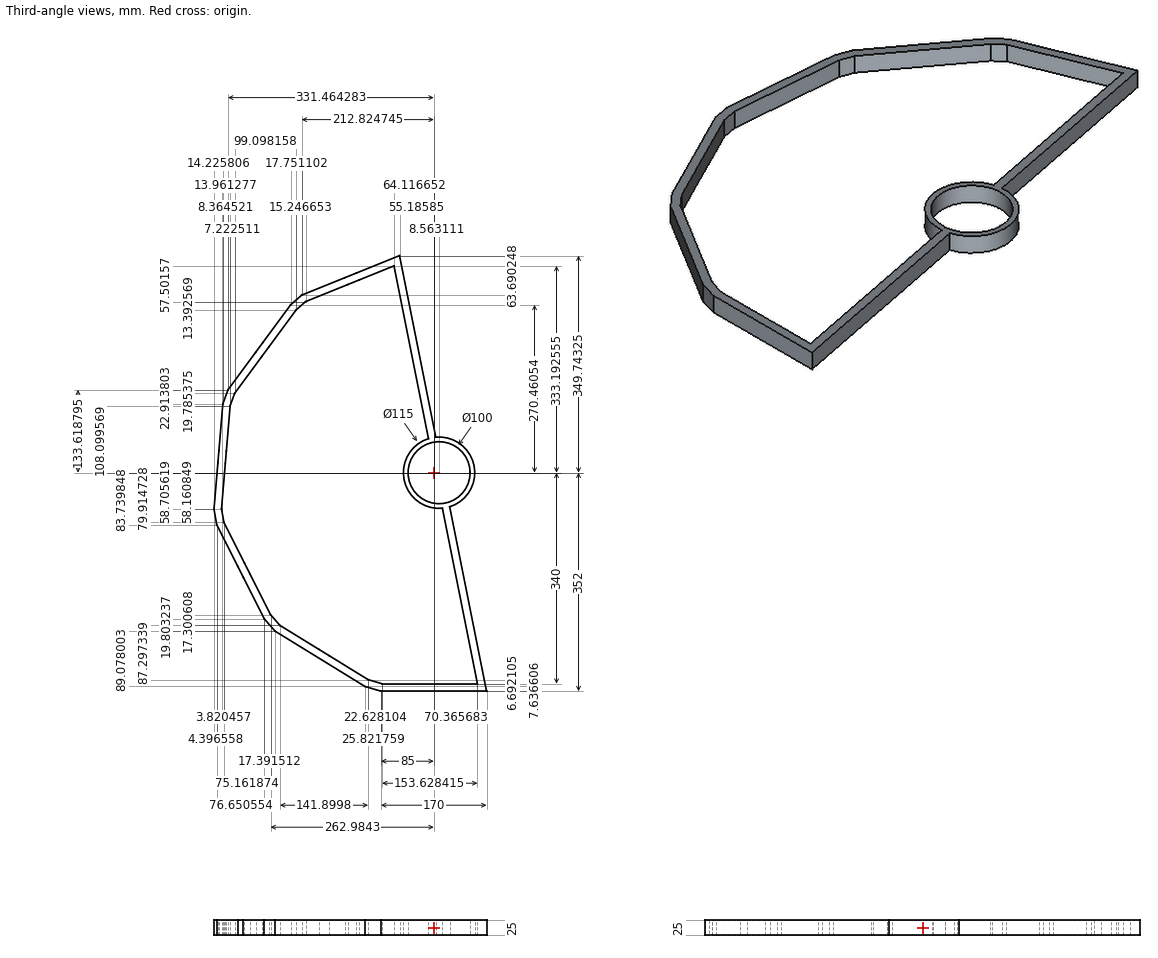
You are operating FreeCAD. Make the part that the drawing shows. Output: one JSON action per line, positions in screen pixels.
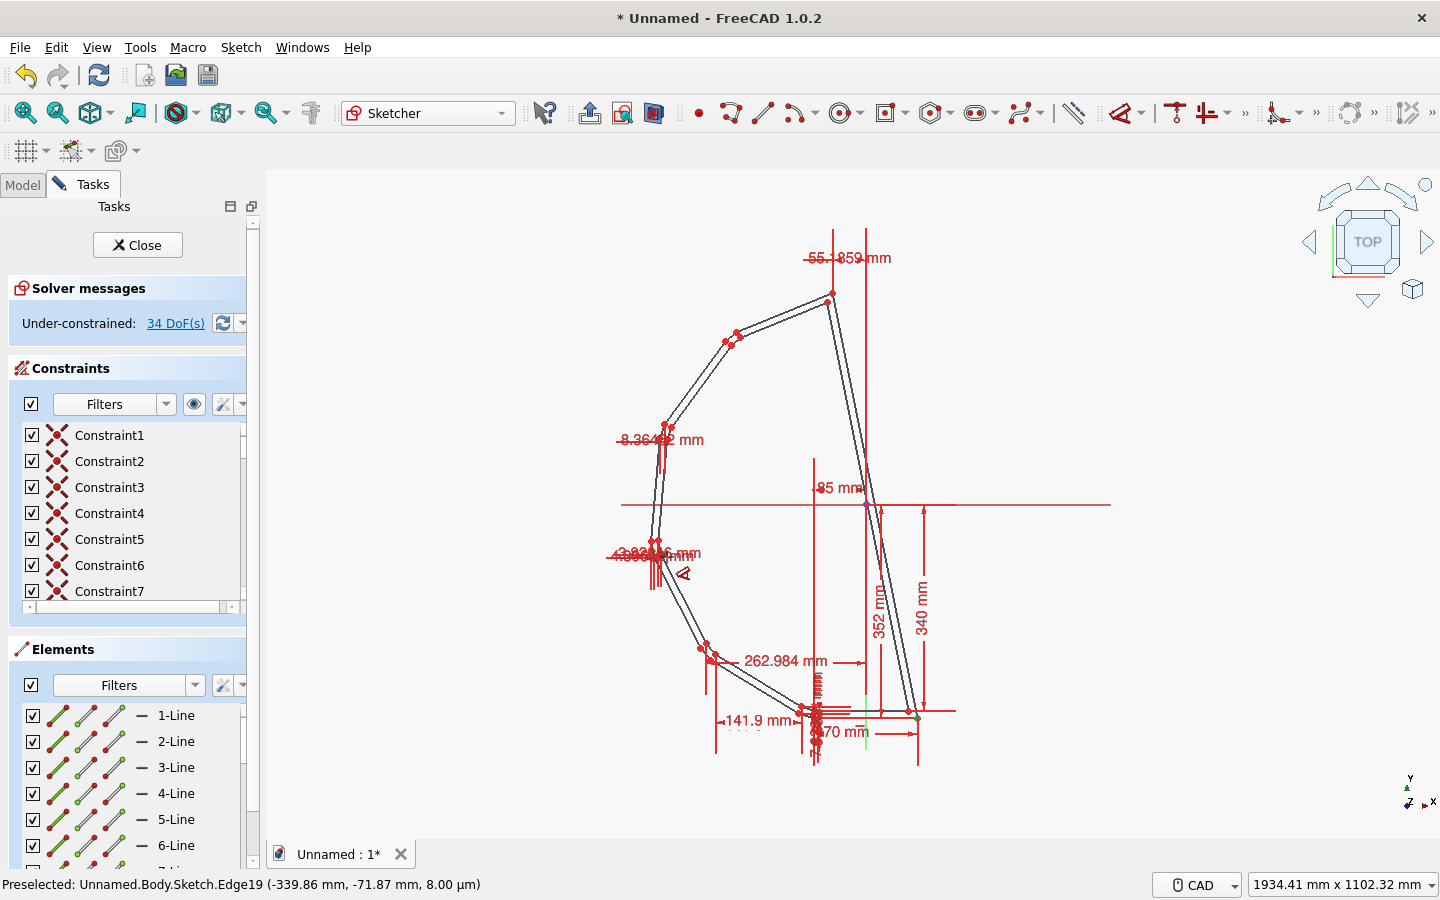
{"action": "scroll", "coordinate": [668, 436], "scroll_direction": "up", "scroll_amount": 12}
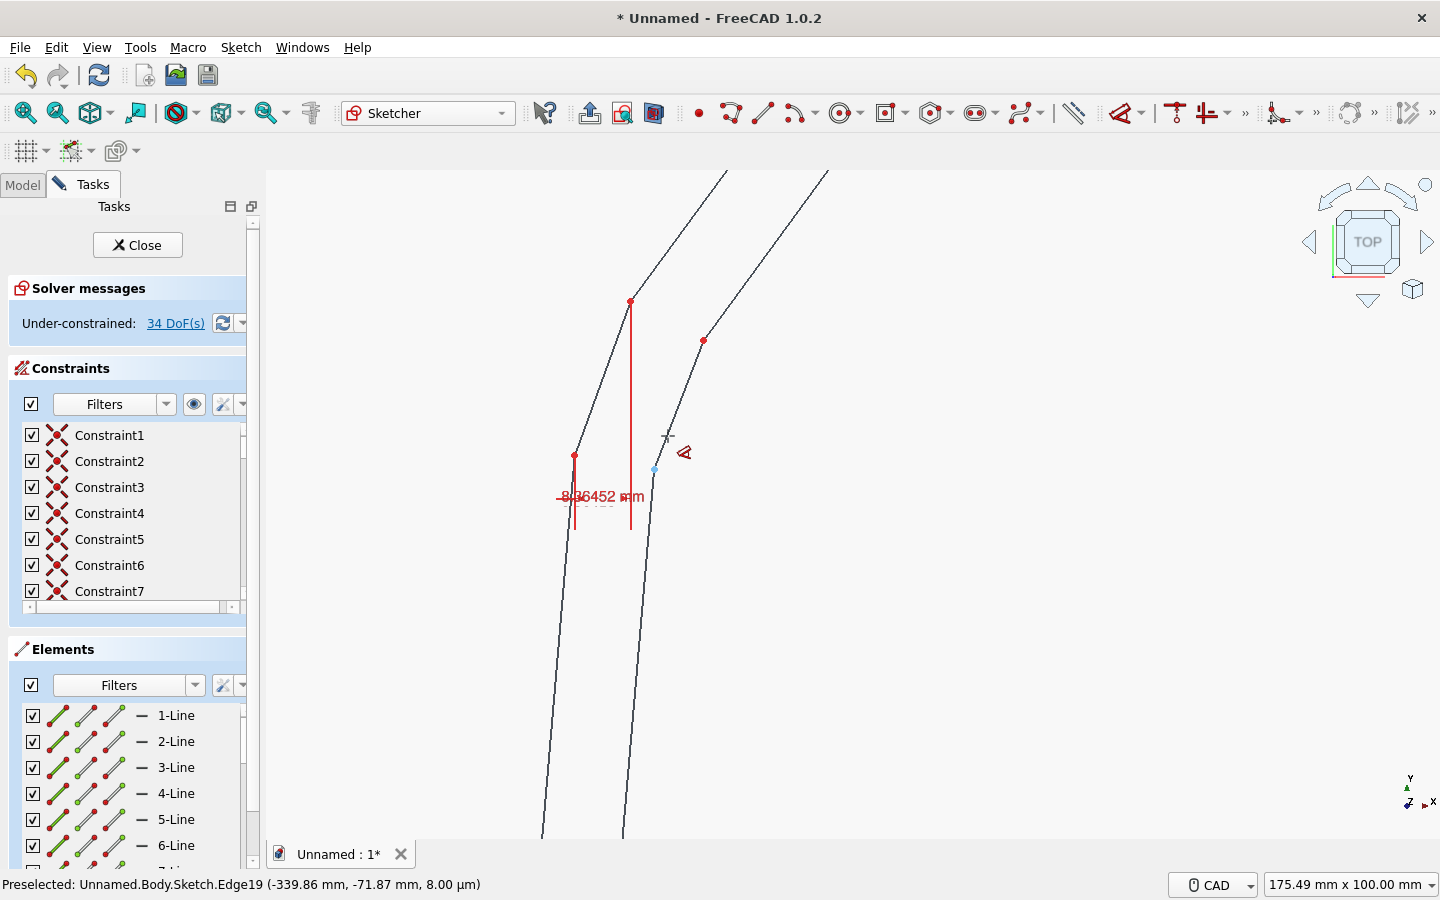
{"action": "left_click", "coordinate": [669, 431]}
{"action": "left_click", "coordinate": [679, 307]}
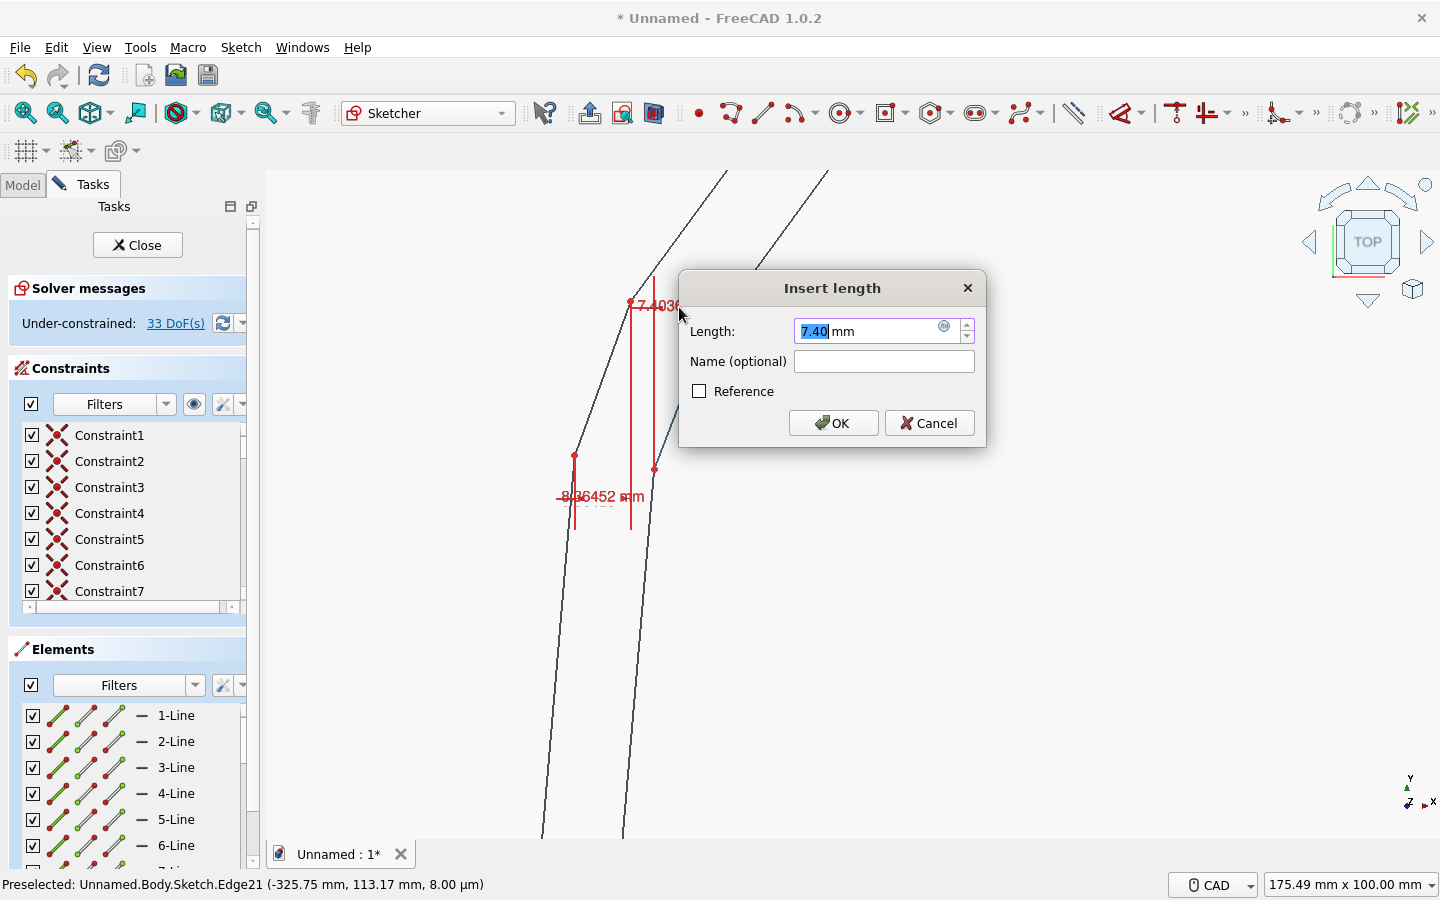
{"action": "type", "text": "7.222511"}
{"action": "key", "text": "Return"}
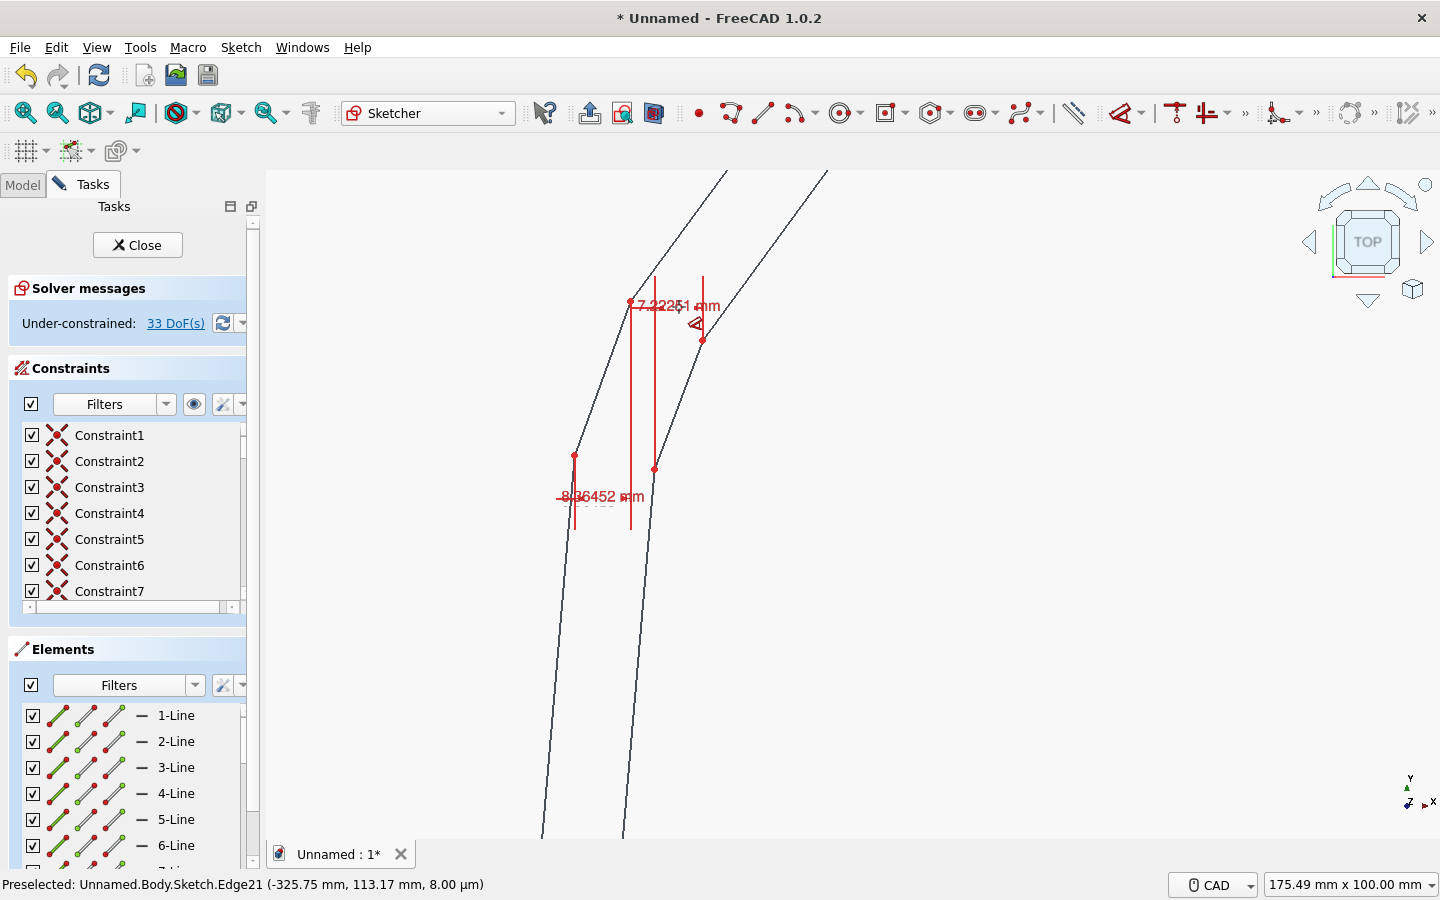
{"action": "scroll", "coordinate": [668, 435], "scroll_direction": "down", "scroll_amount": 12}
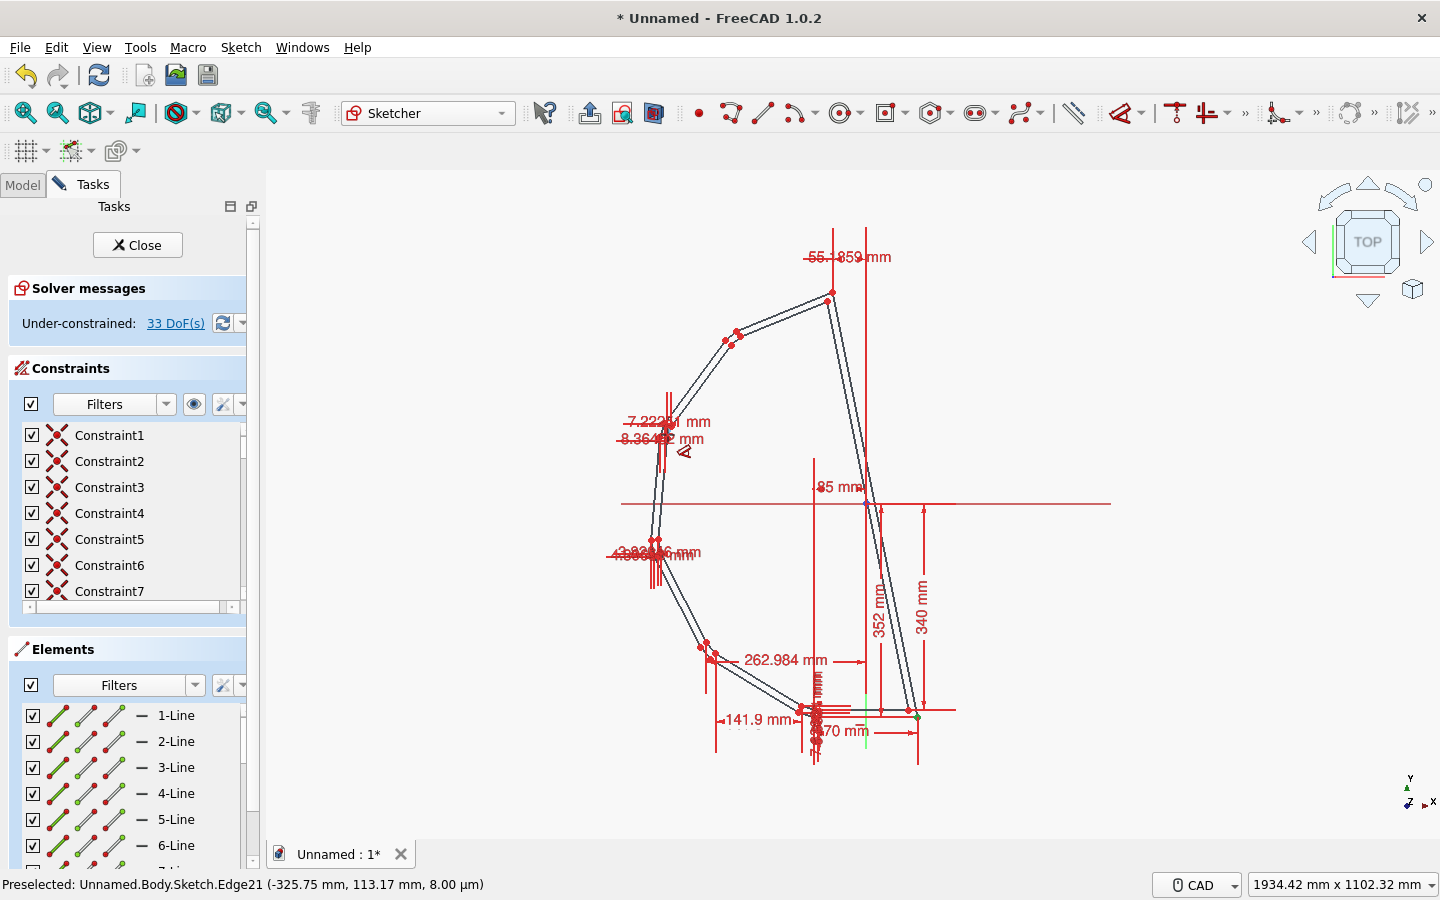
{"action": "scroll", "coordinate": [767, 326], "scroll_direction": "up", "scroll_amount": 4}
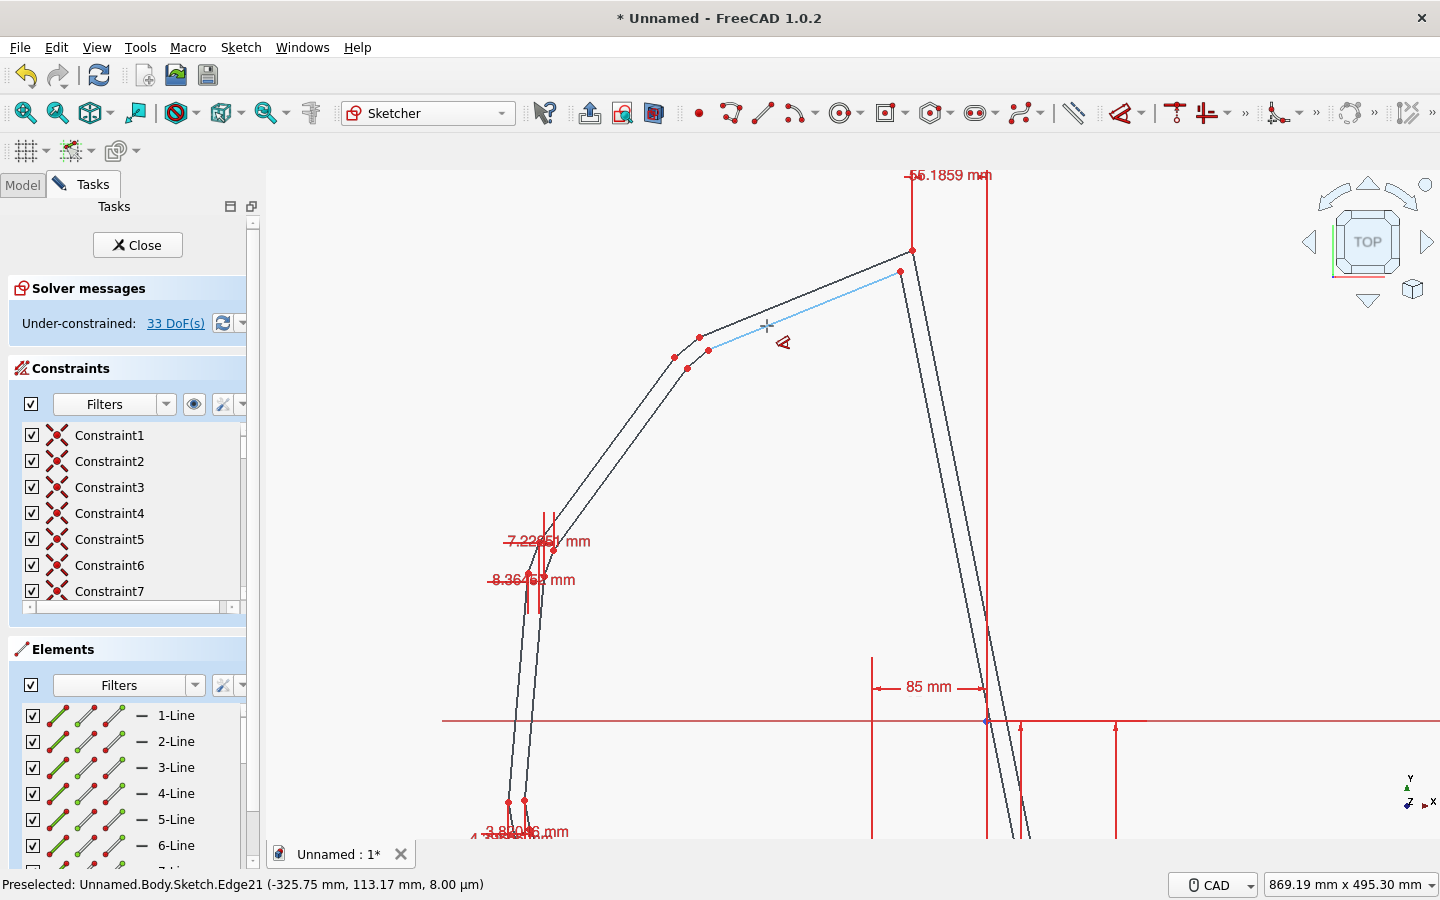
{"action": "left_click", "coordinate": [766, 327]}
{"action": "left_click", "coordinate": [674, 311]}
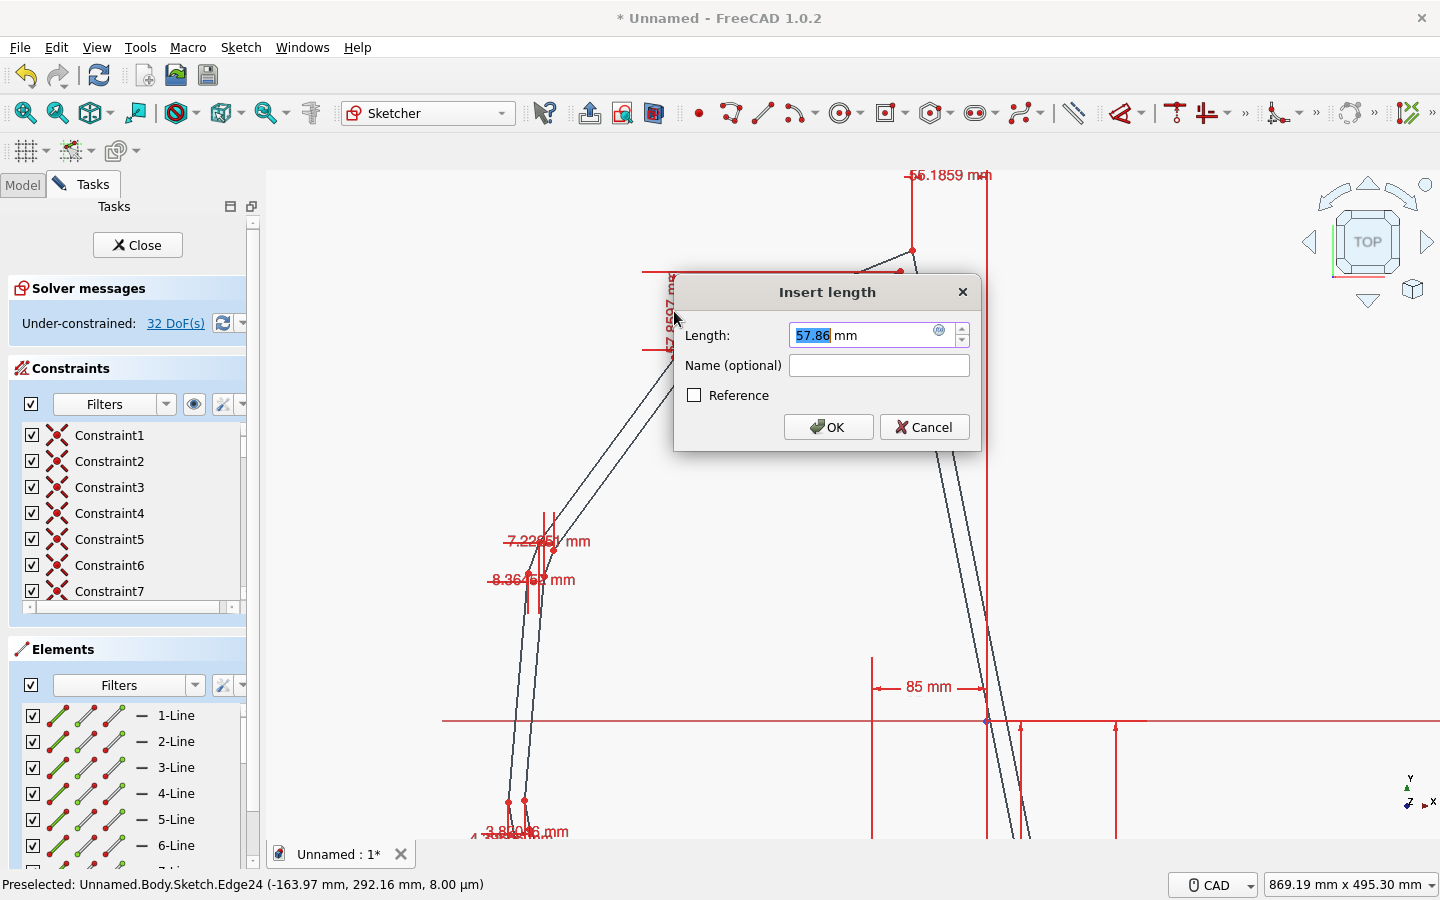
{"action": "type", "text": "57.50157"}
{"action": "key", "text": "Return"}